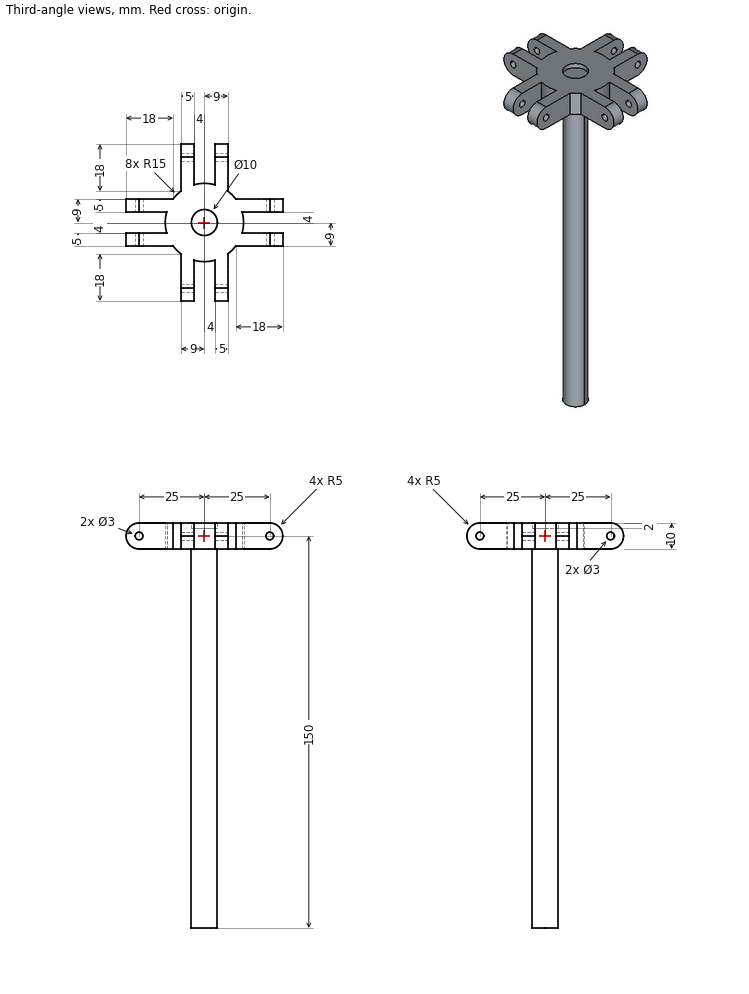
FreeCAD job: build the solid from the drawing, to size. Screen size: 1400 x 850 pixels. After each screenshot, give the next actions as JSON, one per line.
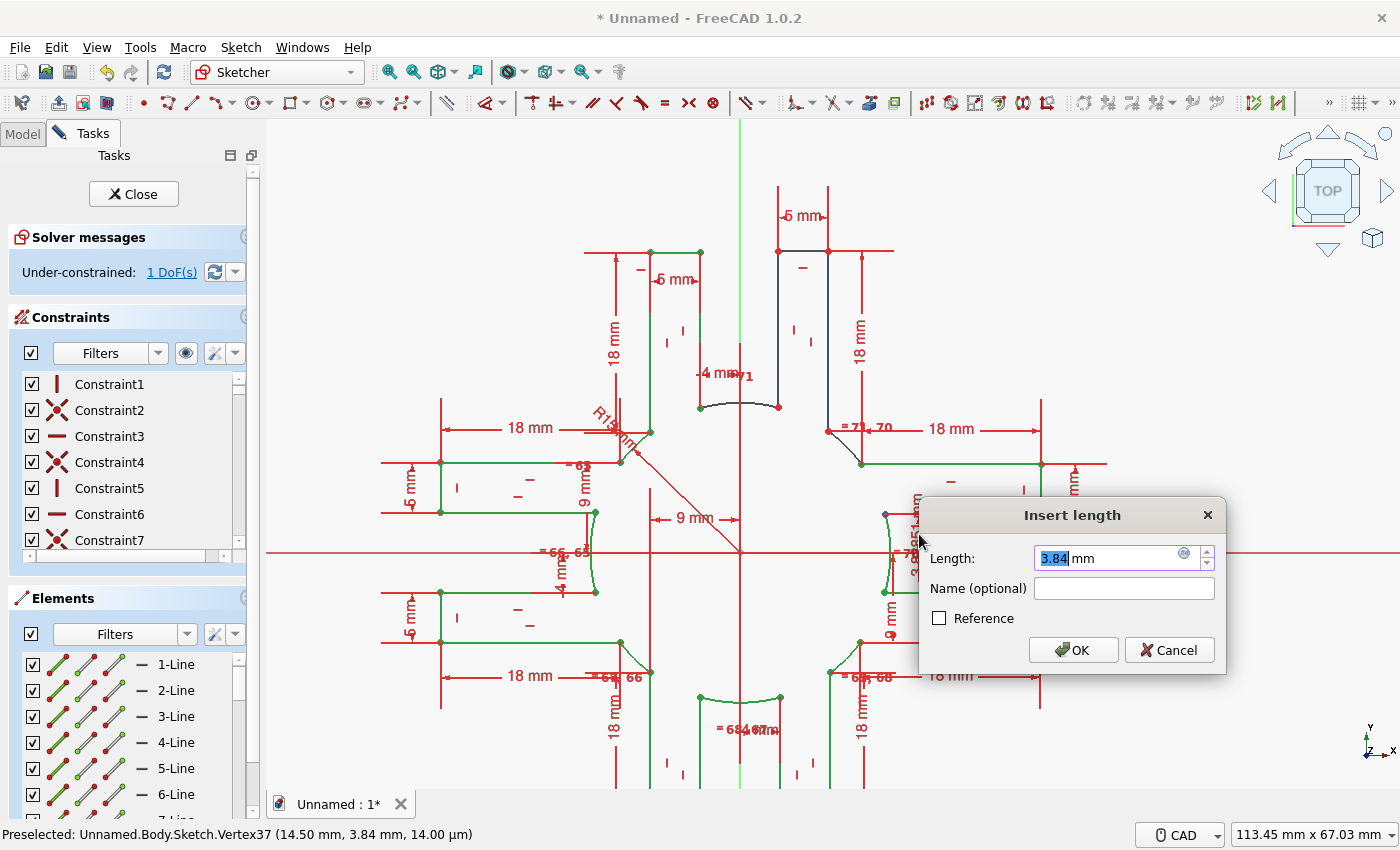
{"action": "type", "text": "4"}
{"action": "key", "text": "Return"}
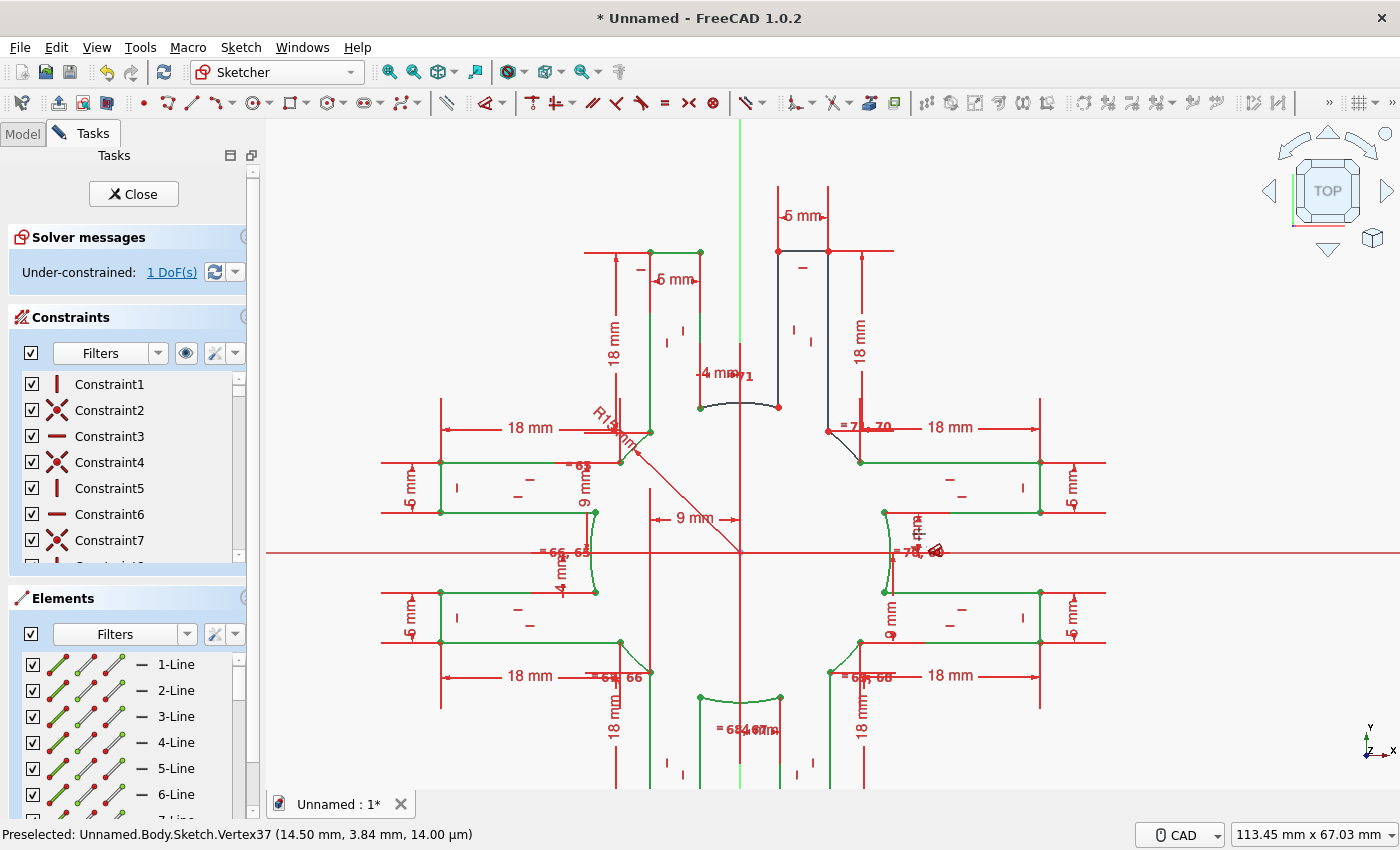
{"action": "left_click", "coordinate": [828, 431]}
{"action": "left_click", "coordinate": [804, 397]}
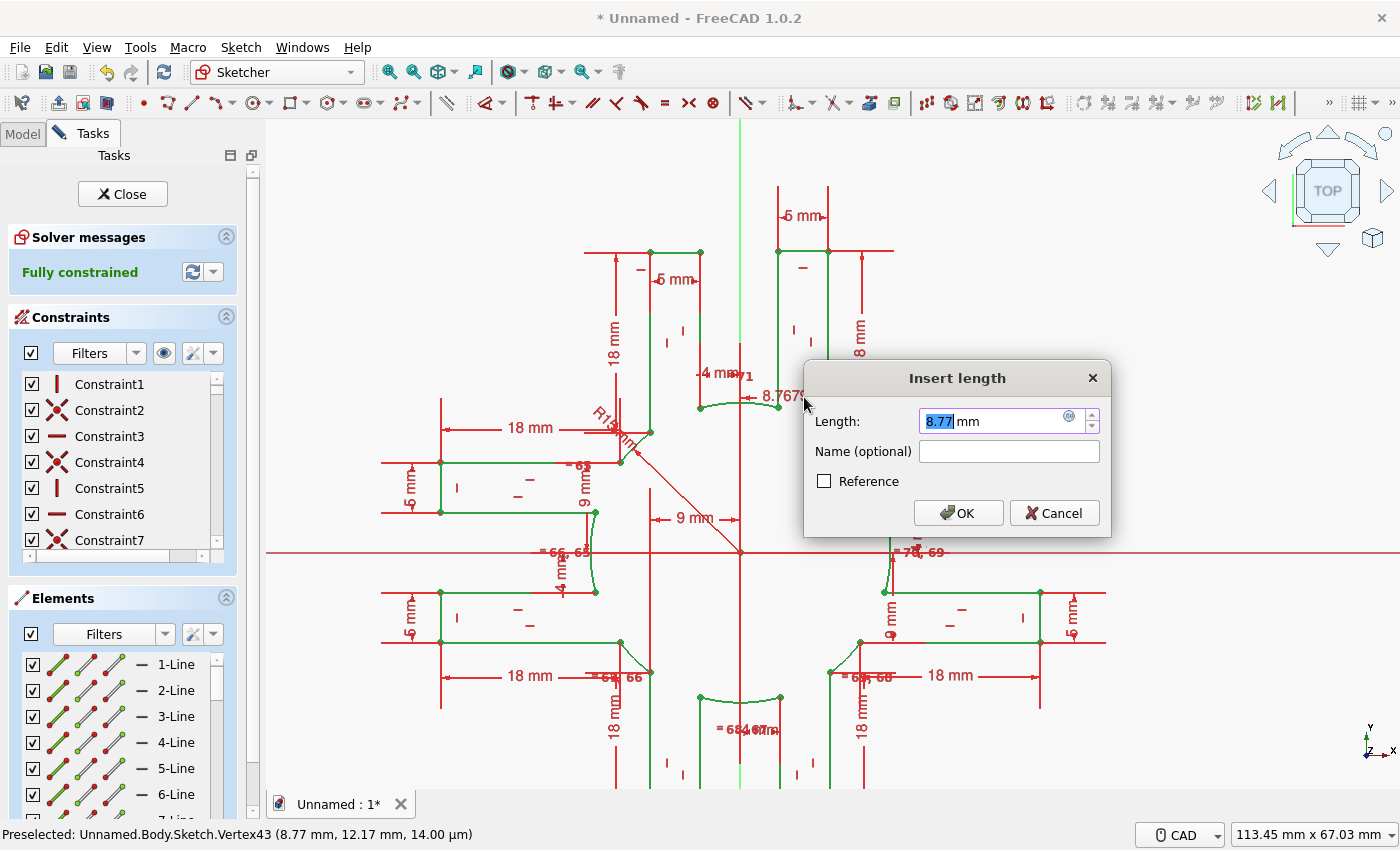
{"action": "type", "text": "9"}
{"action": "key", "text": "Return"}
{"action": "key", "text": "Escape"}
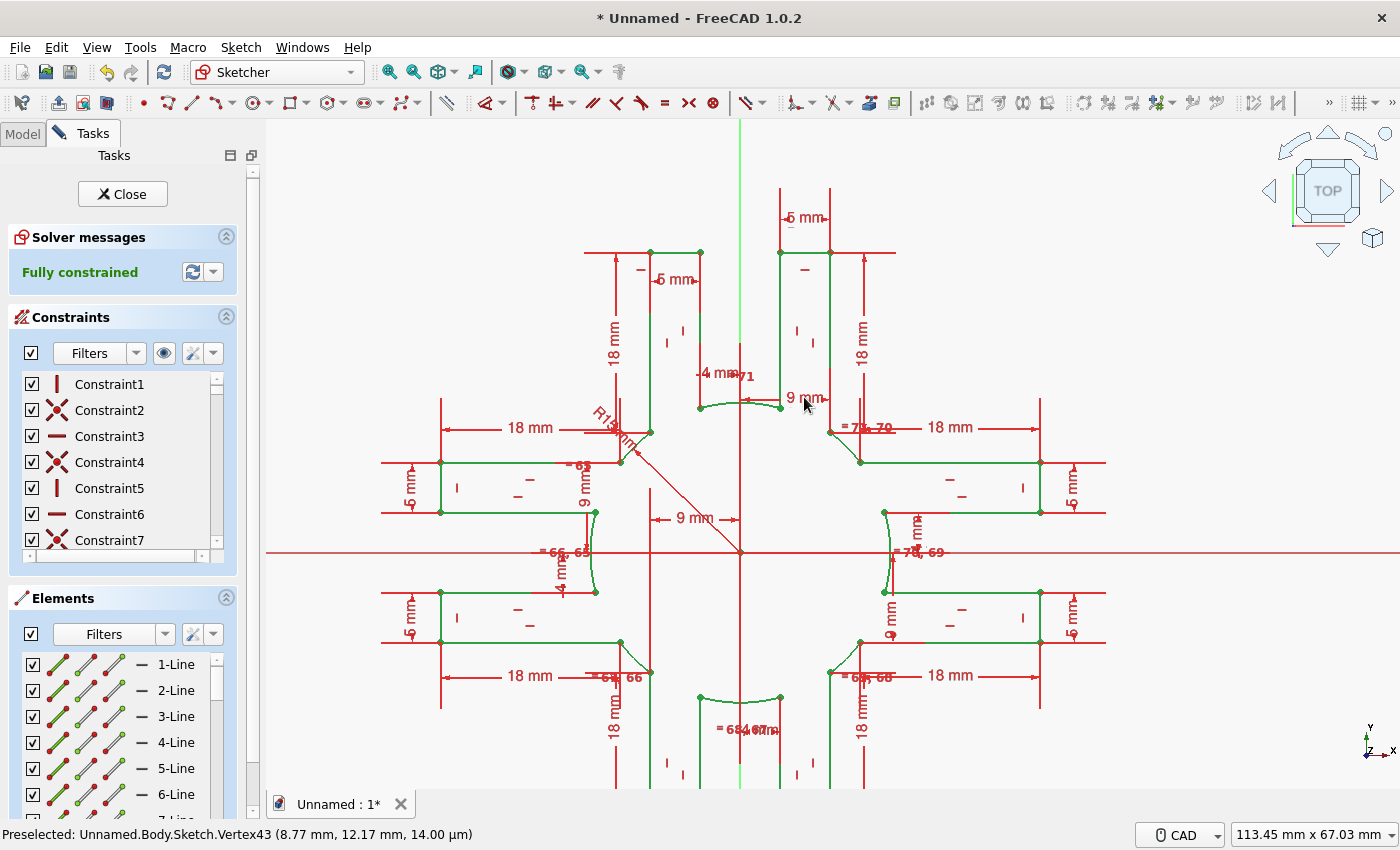
{"action": "left_click", "coordinate": [123, 194]}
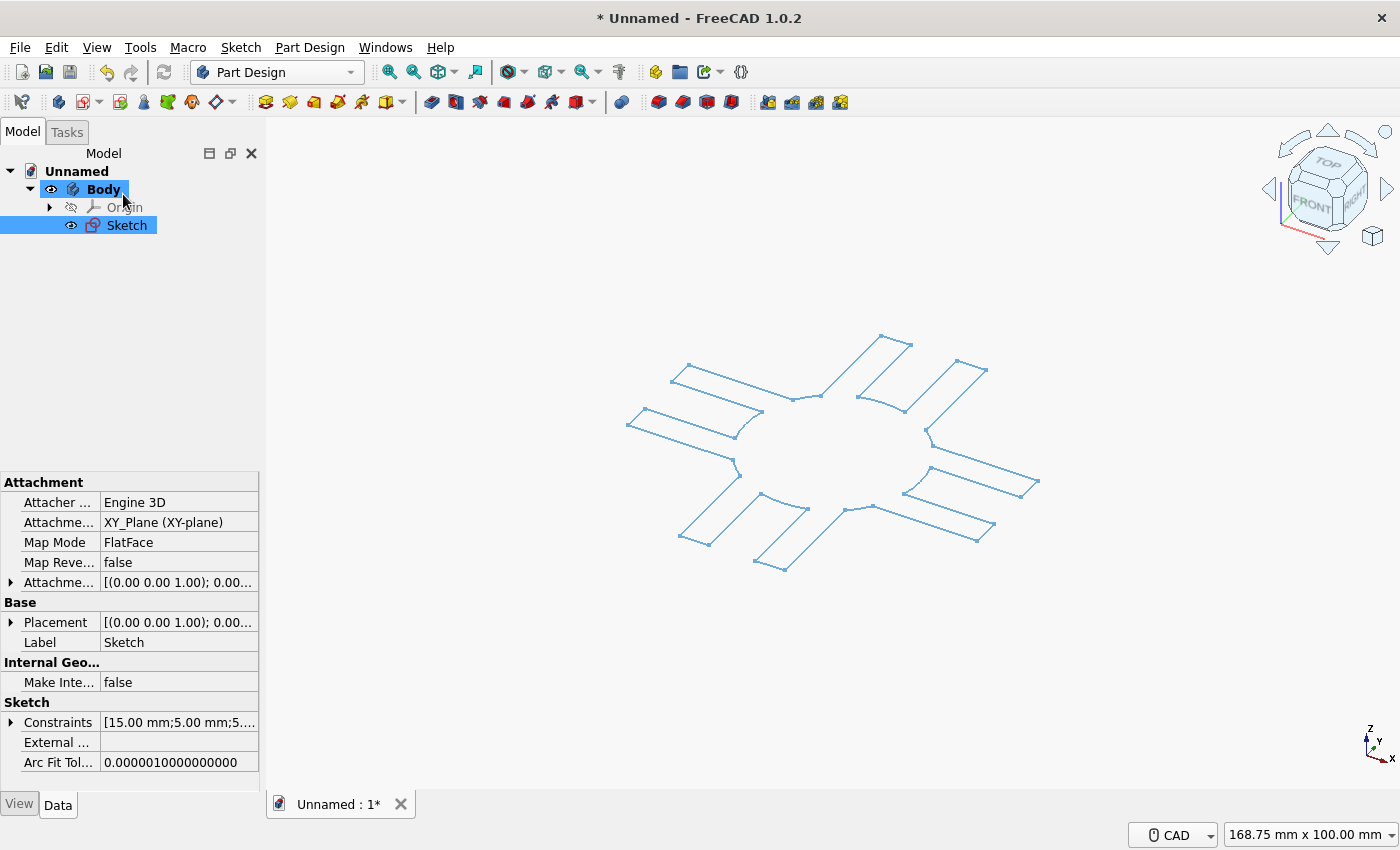
{"action": "left_click", "coordinate": [266, 102]}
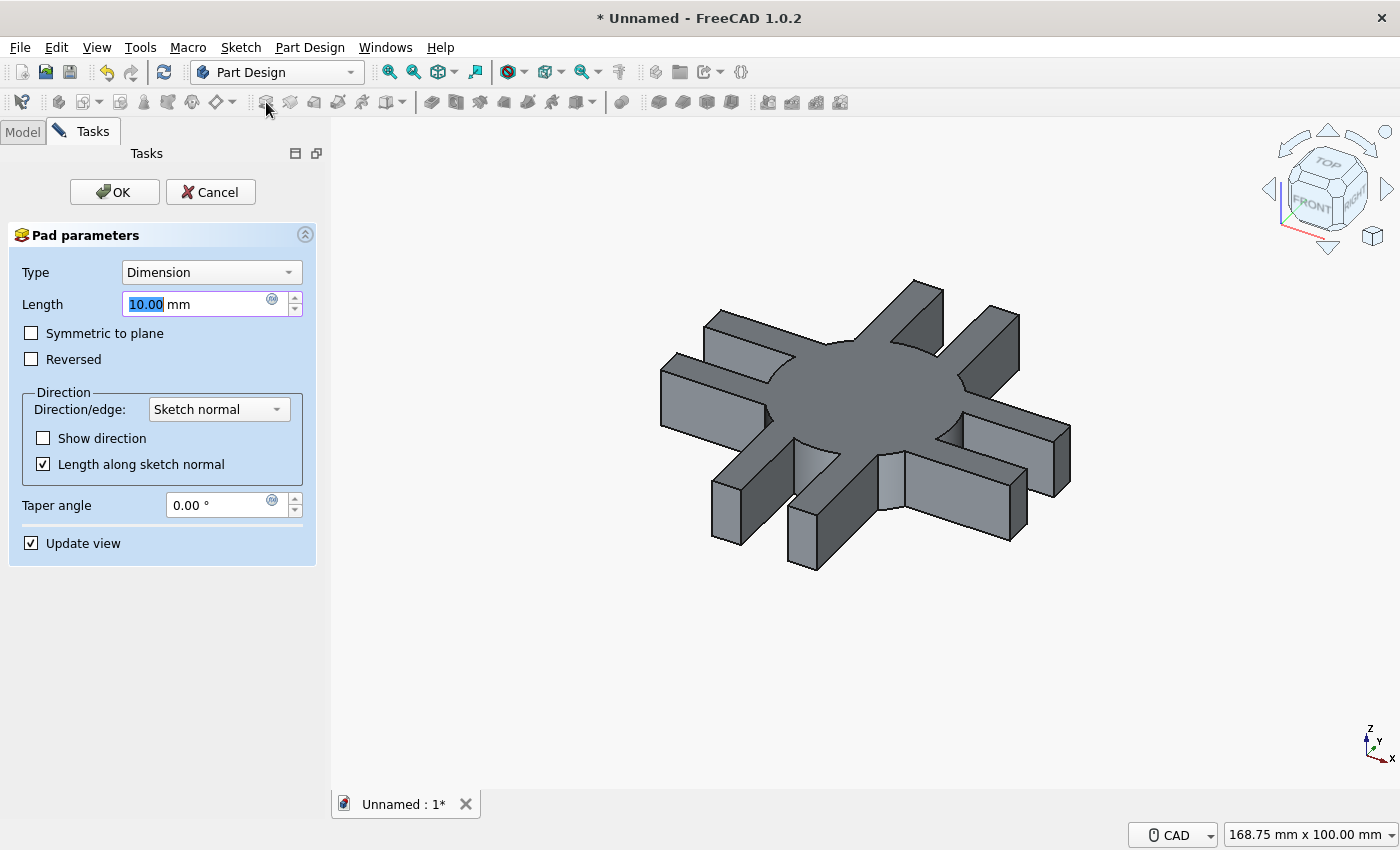
{"action": "type", "text": "10"}
{"action": "key", "text": "Tab"}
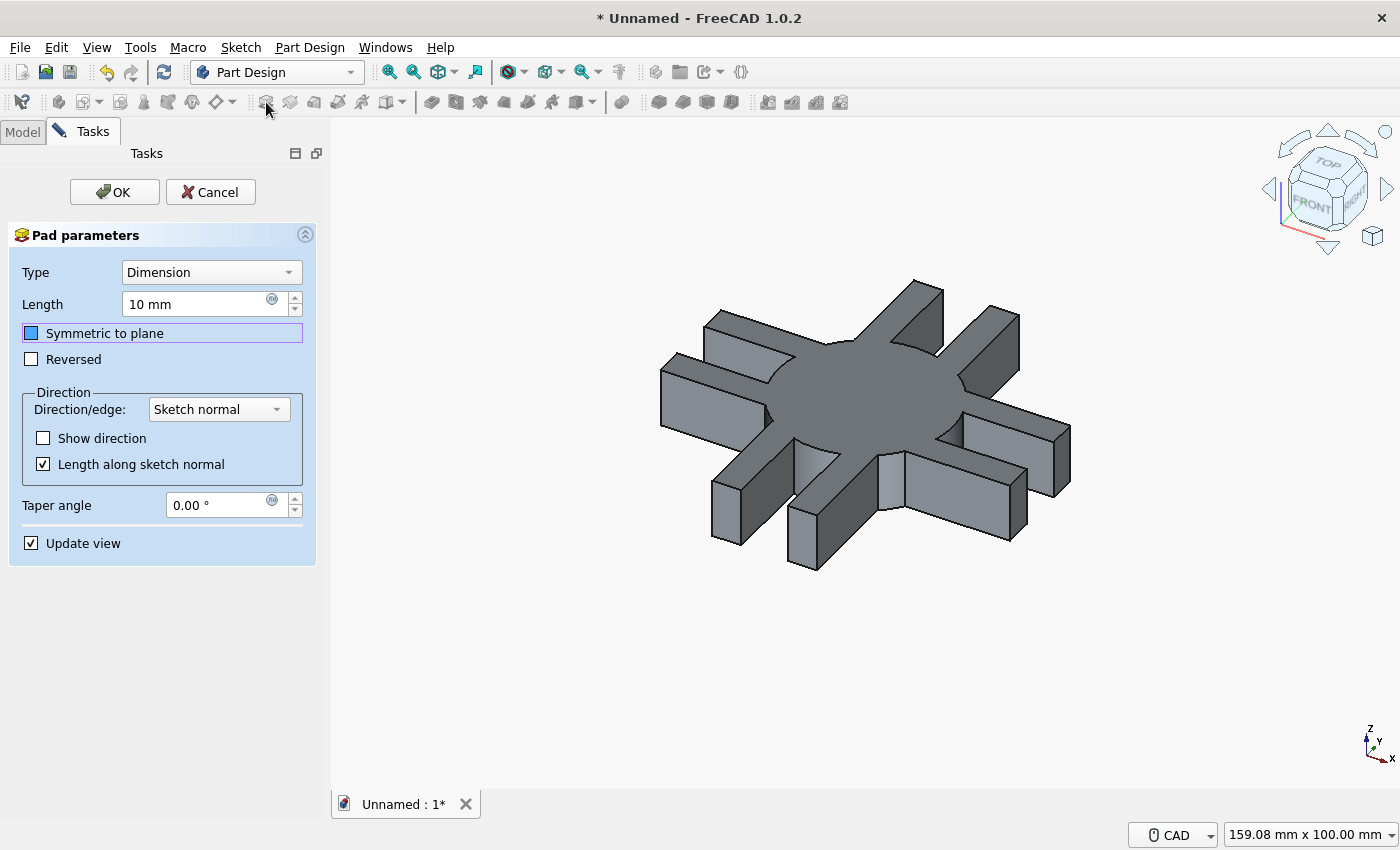
{"action": "left_click", "coordinate": [30, 333]}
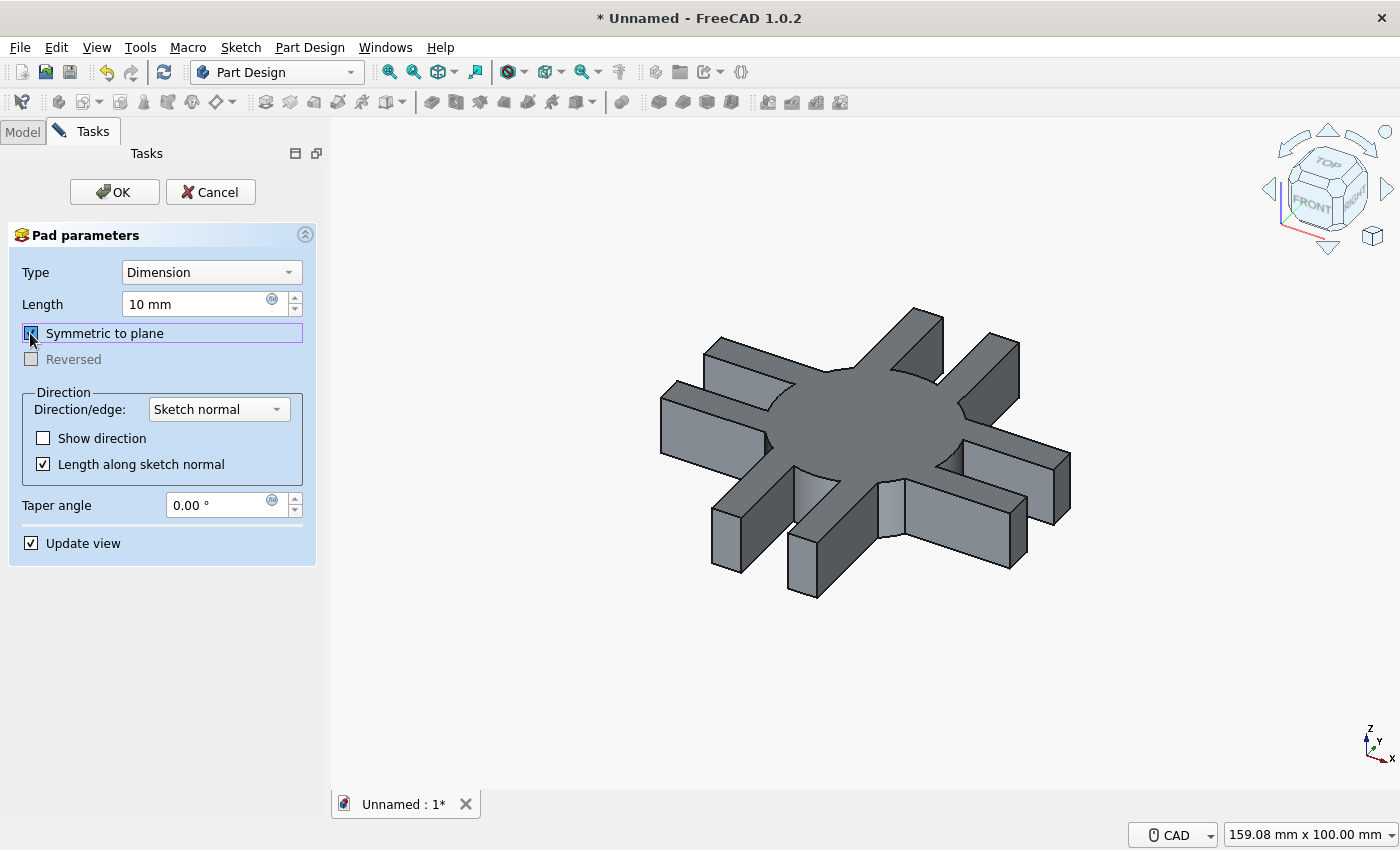
{"action": "left_click", "coordinate": [115, 192]}